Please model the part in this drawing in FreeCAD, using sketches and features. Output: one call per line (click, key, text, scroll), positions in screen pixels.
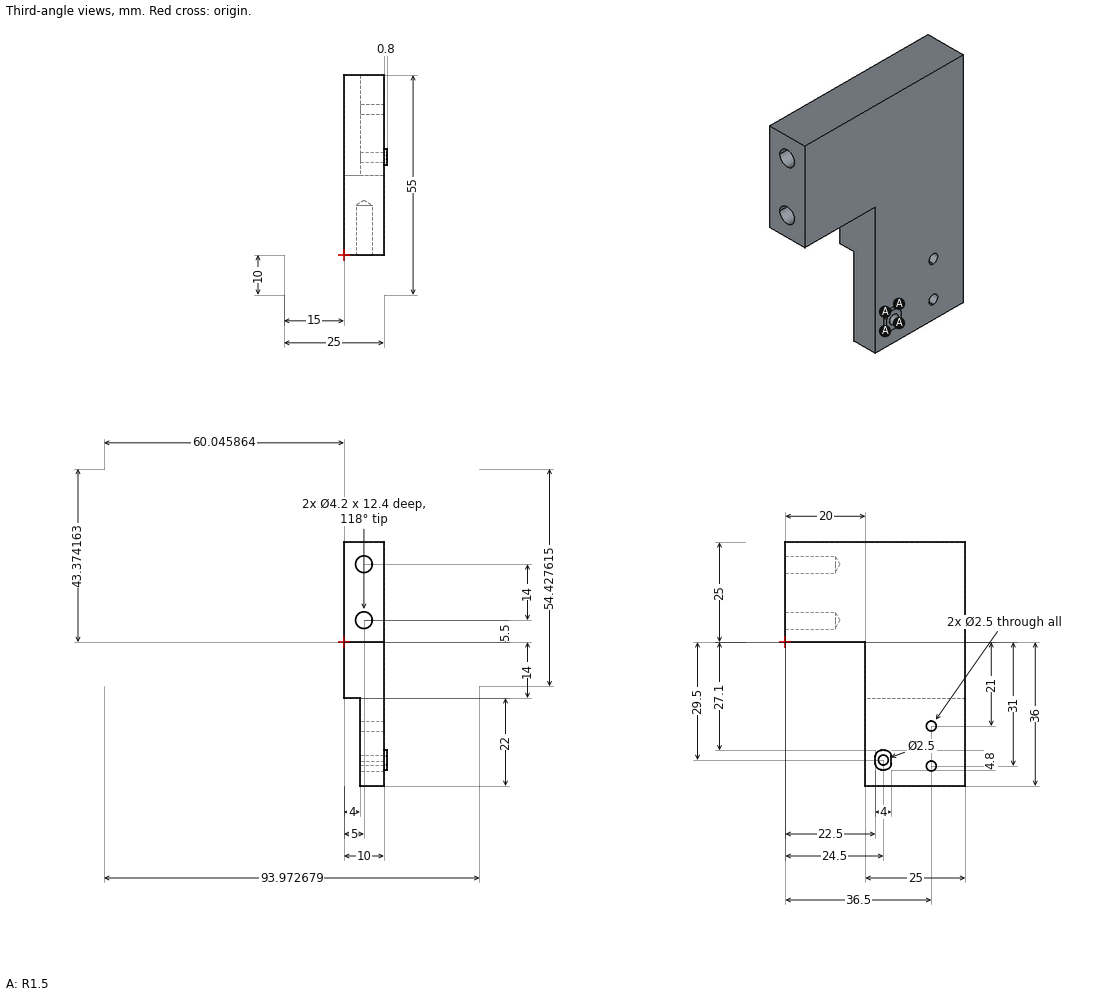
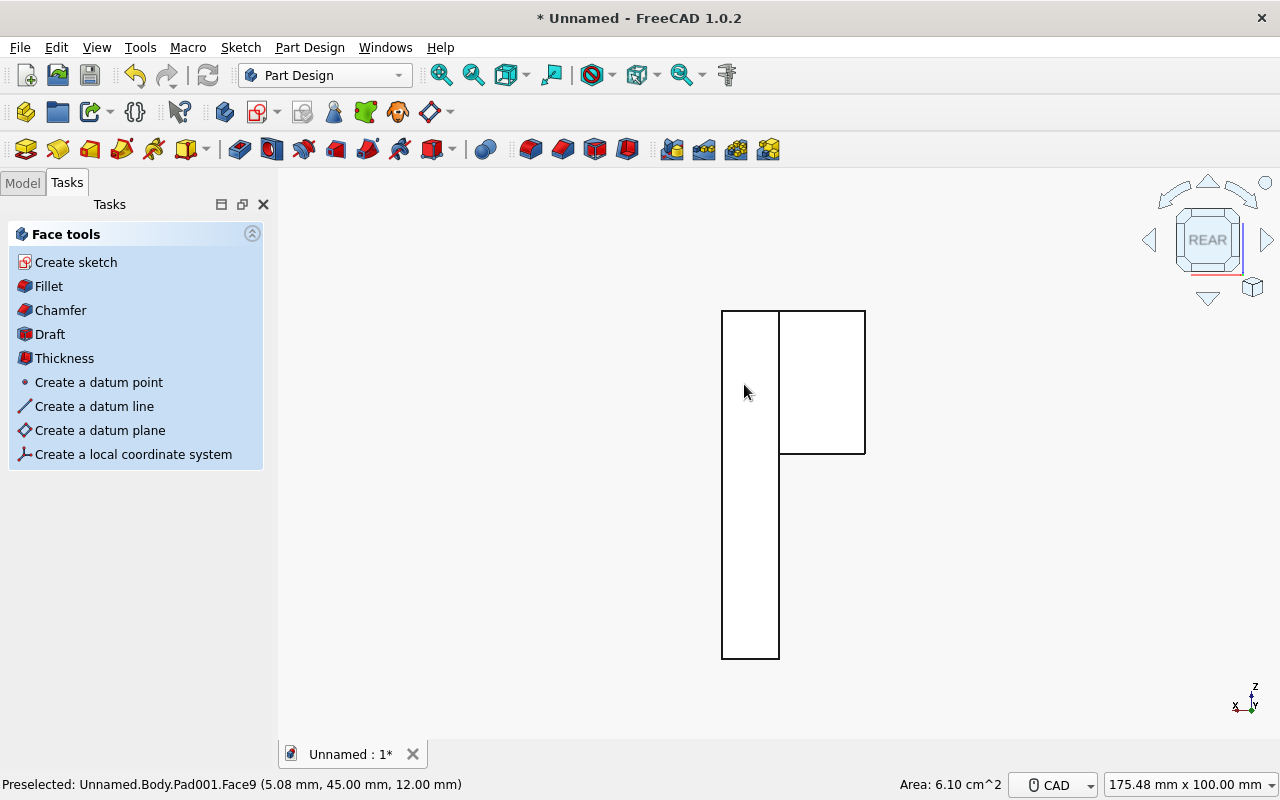
click(258, 112)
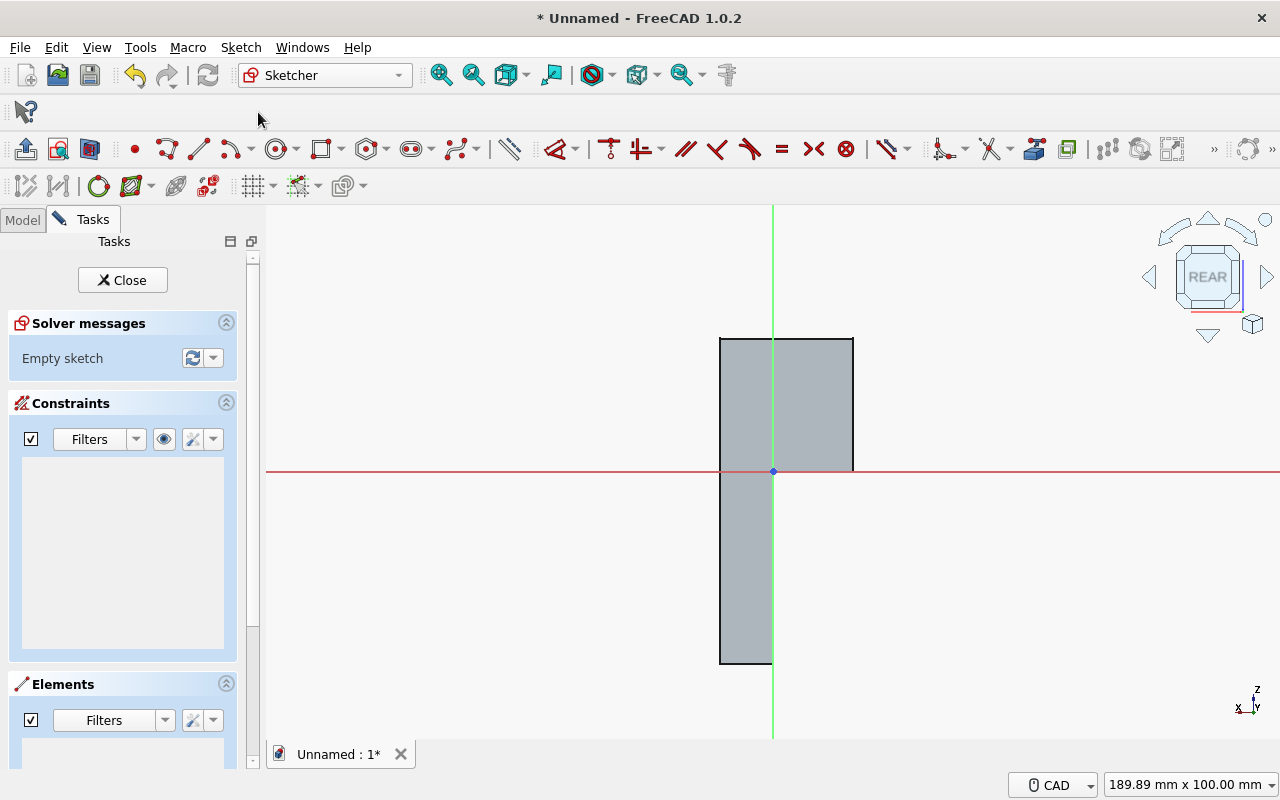
scroll(833, 685, up, 3)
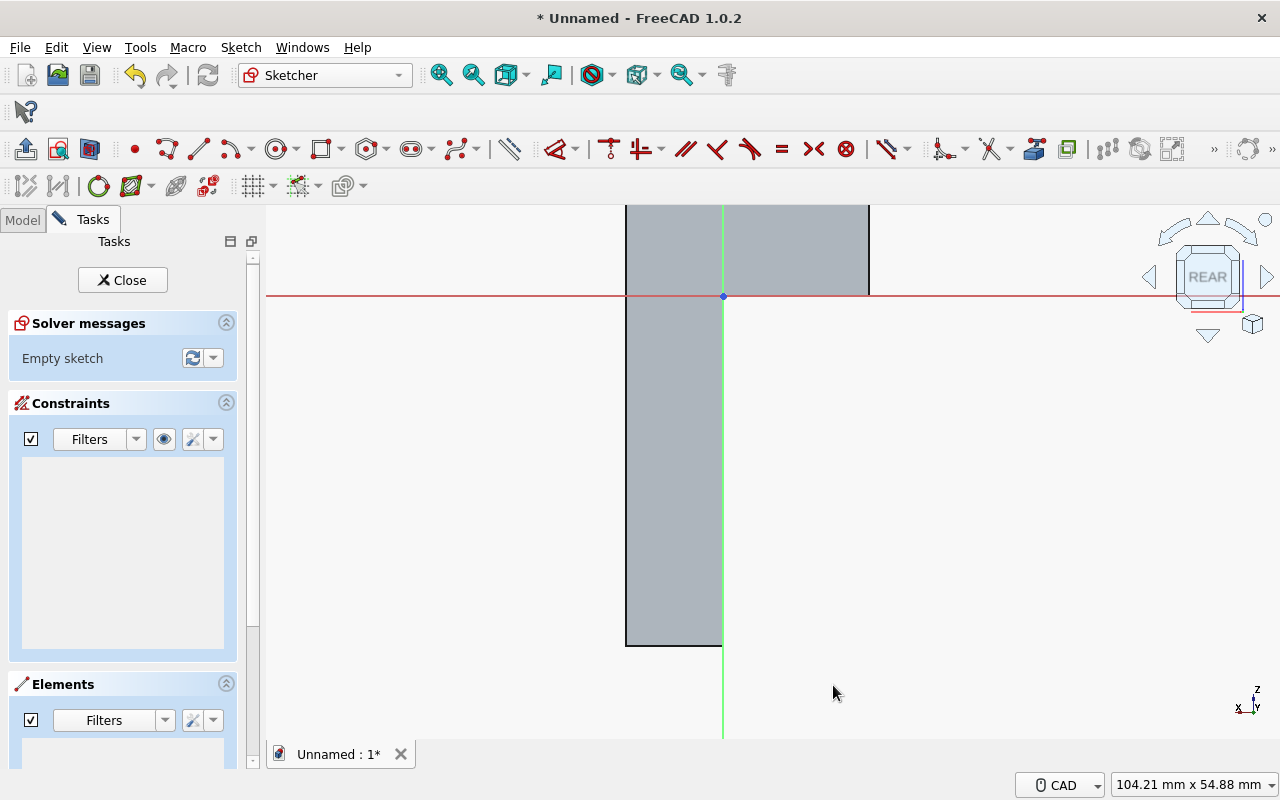
click(322, 150)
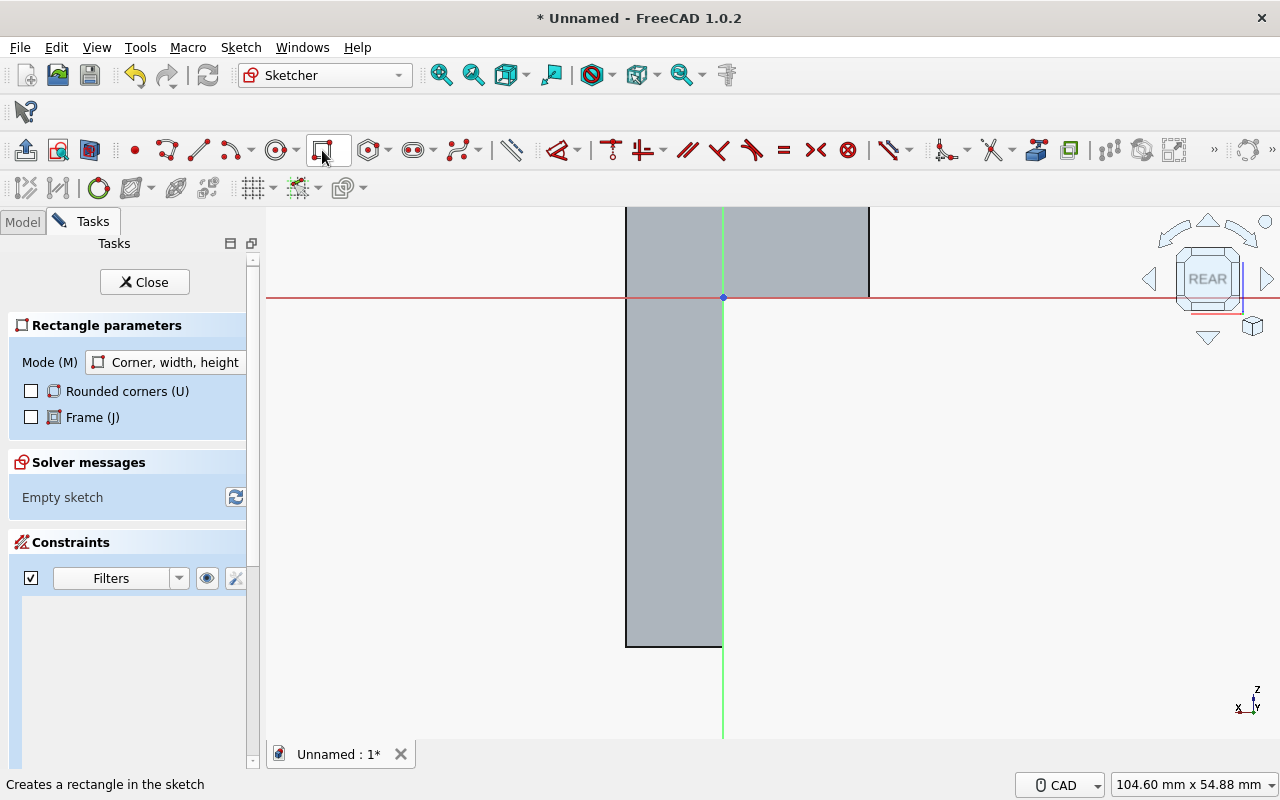
click(685, 434)
click(723, 647)
key(Escape)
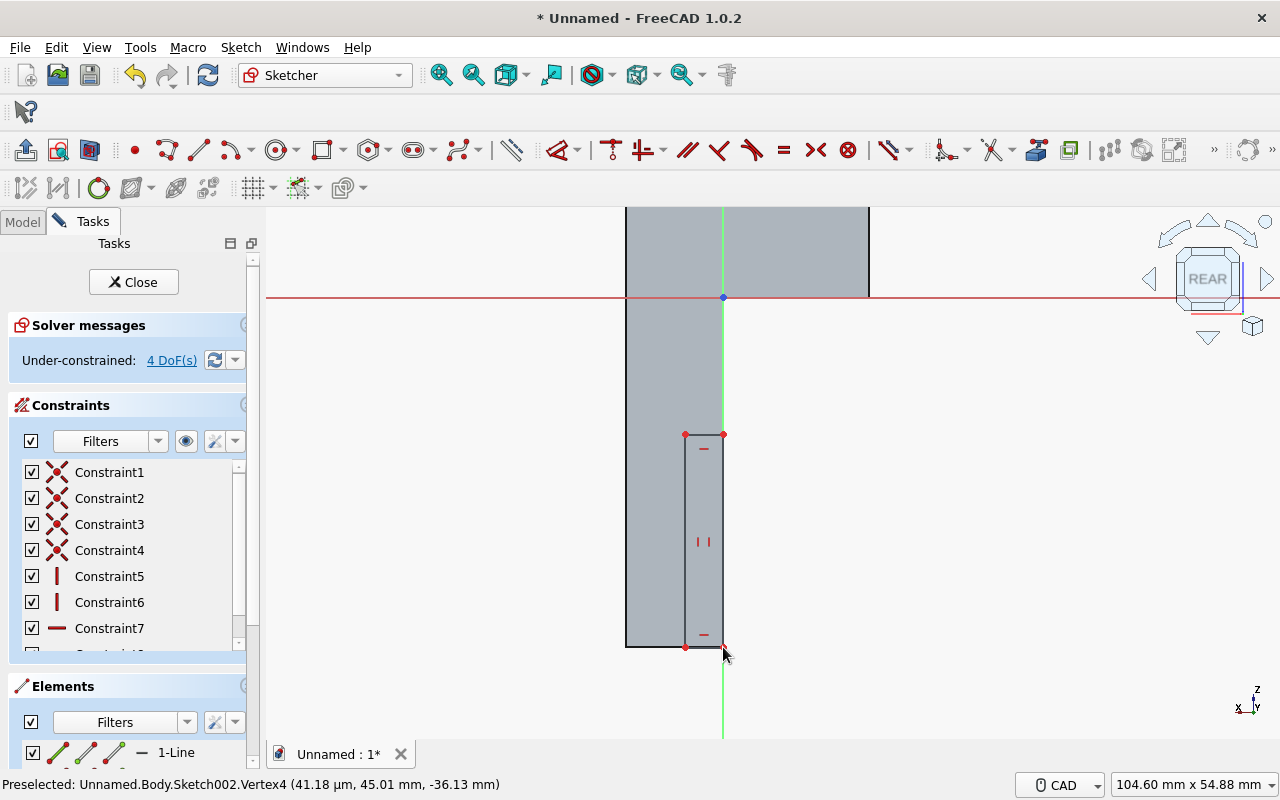
click(723, 648)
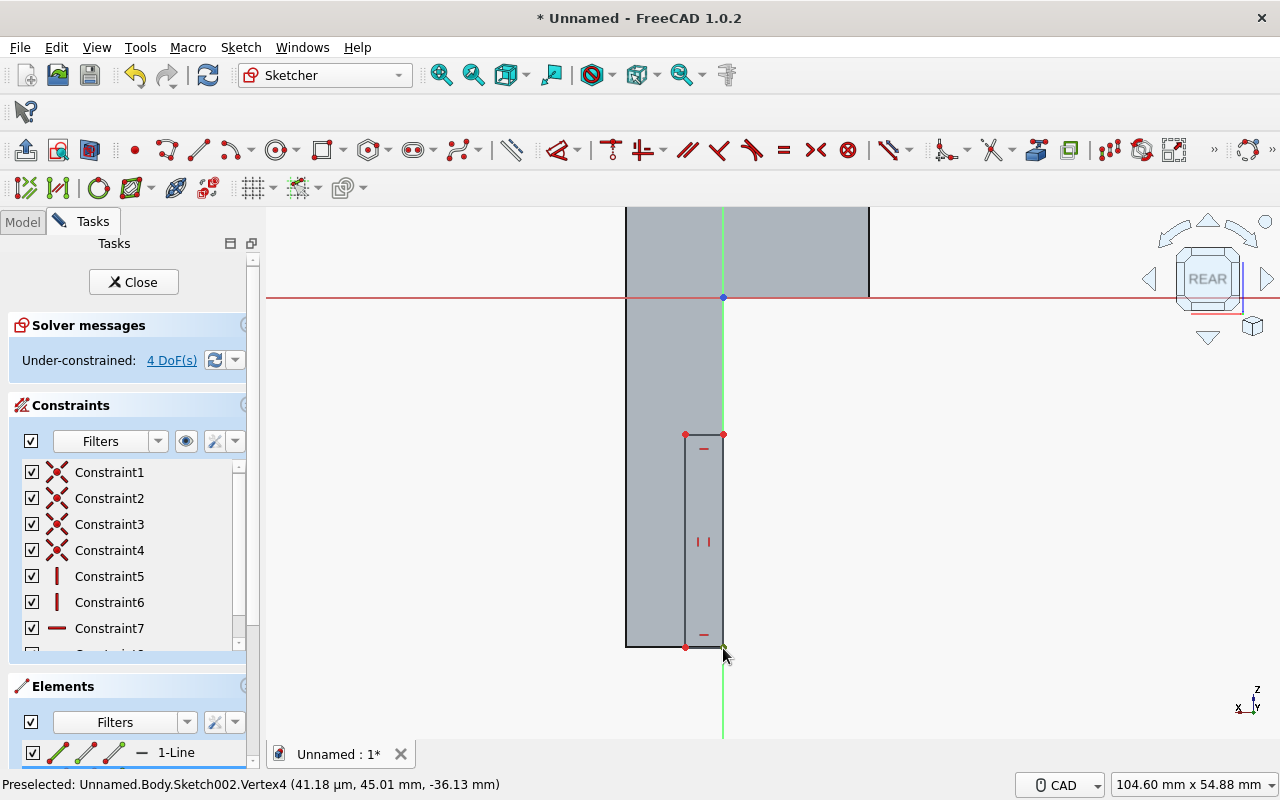
click(723, 405)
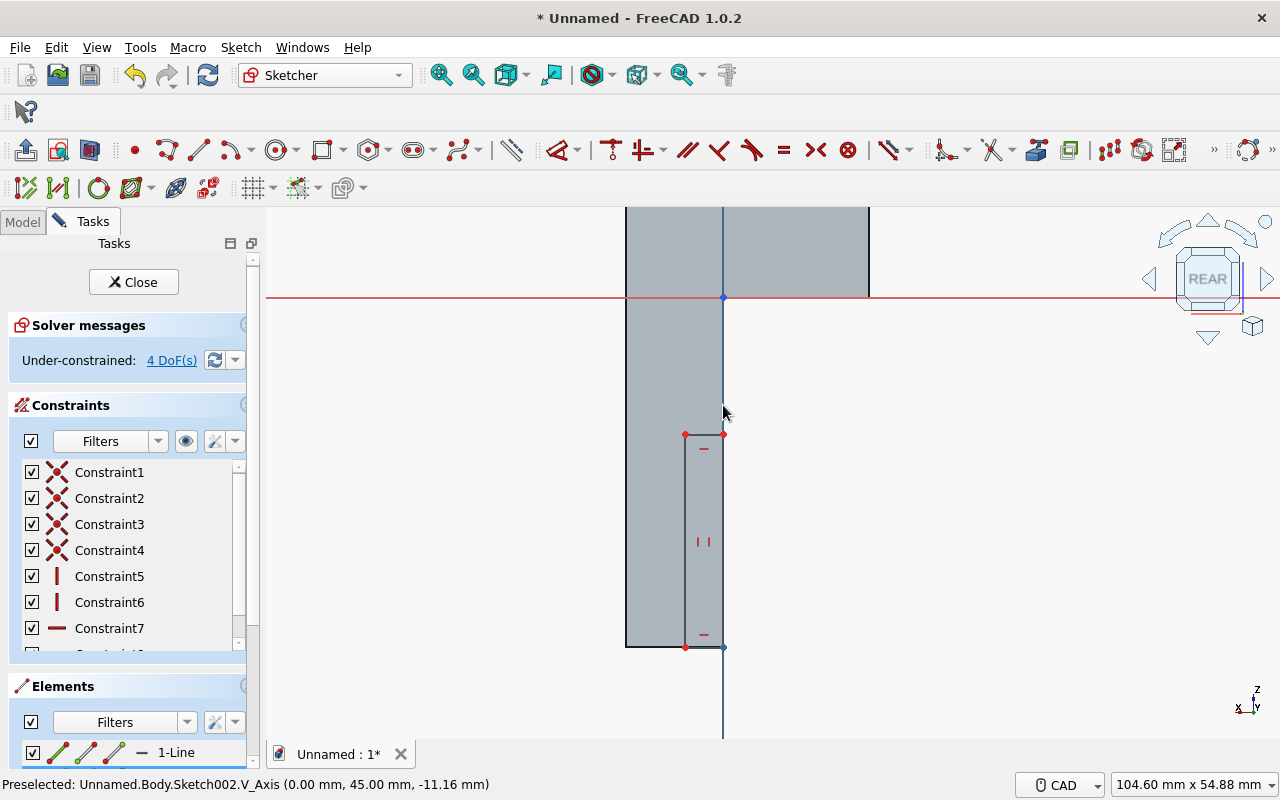
click(612, 150)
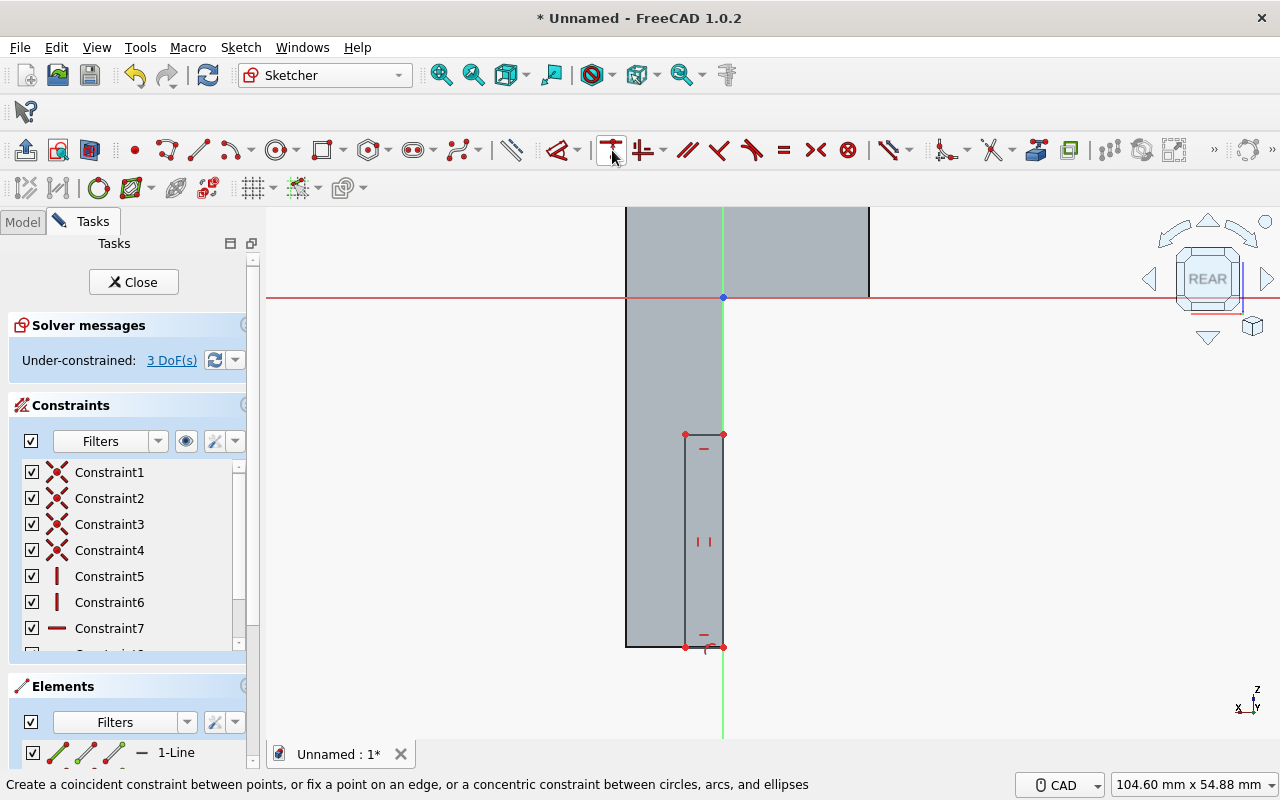
click(558, 150)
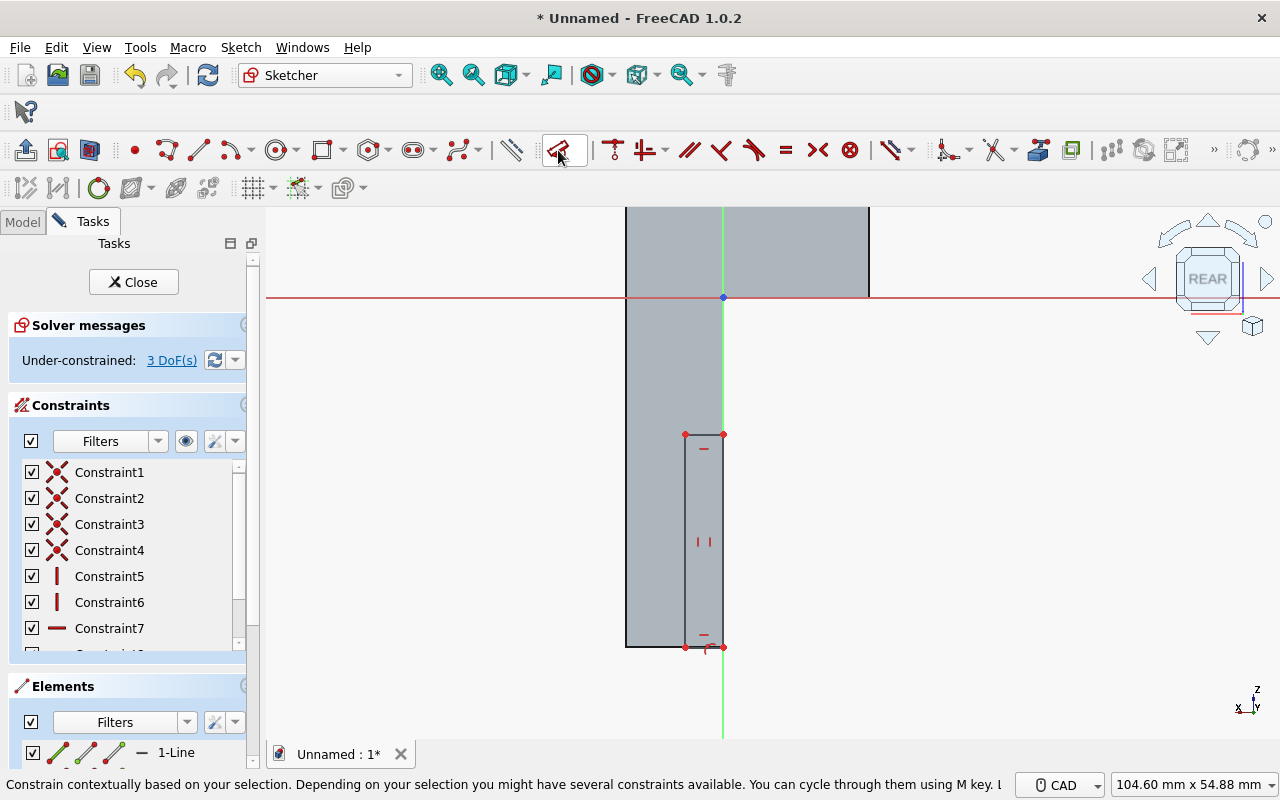
click(697, 648)
click(704, 682)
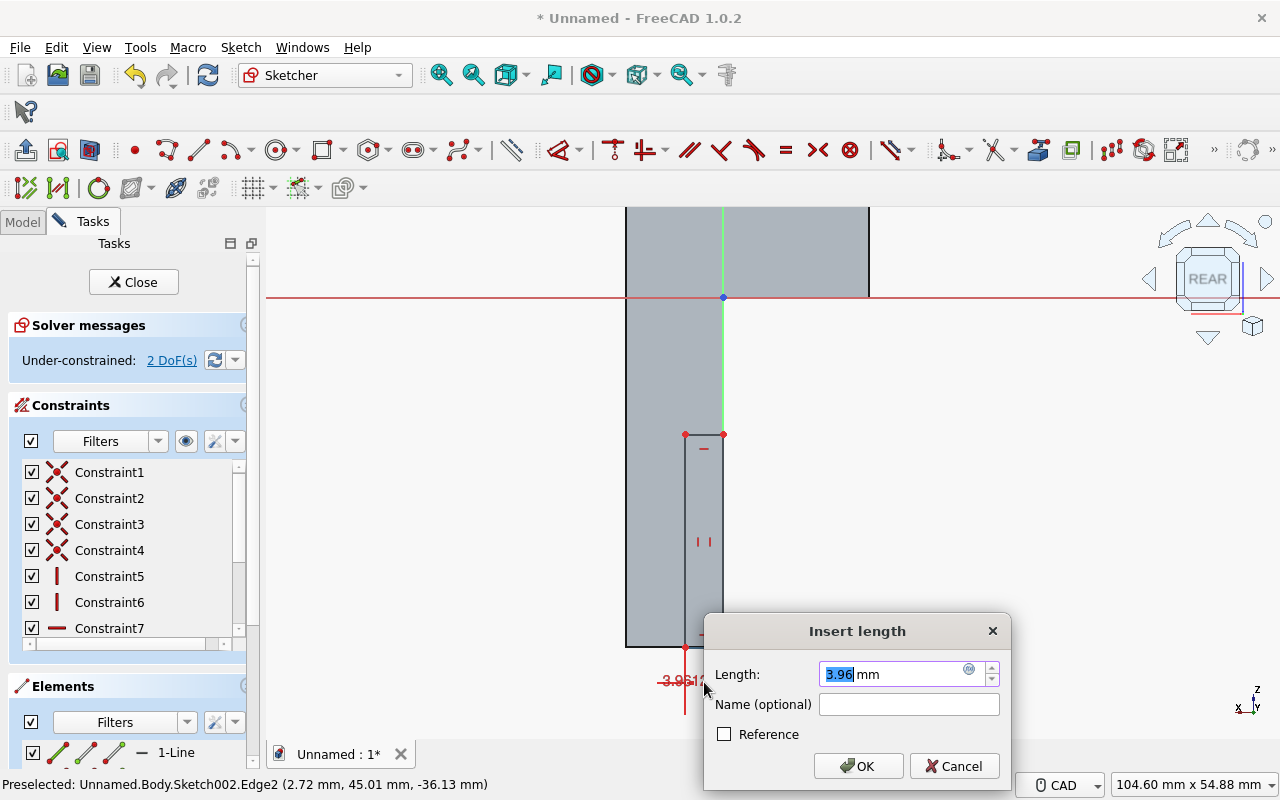
text(4)
key(Return)